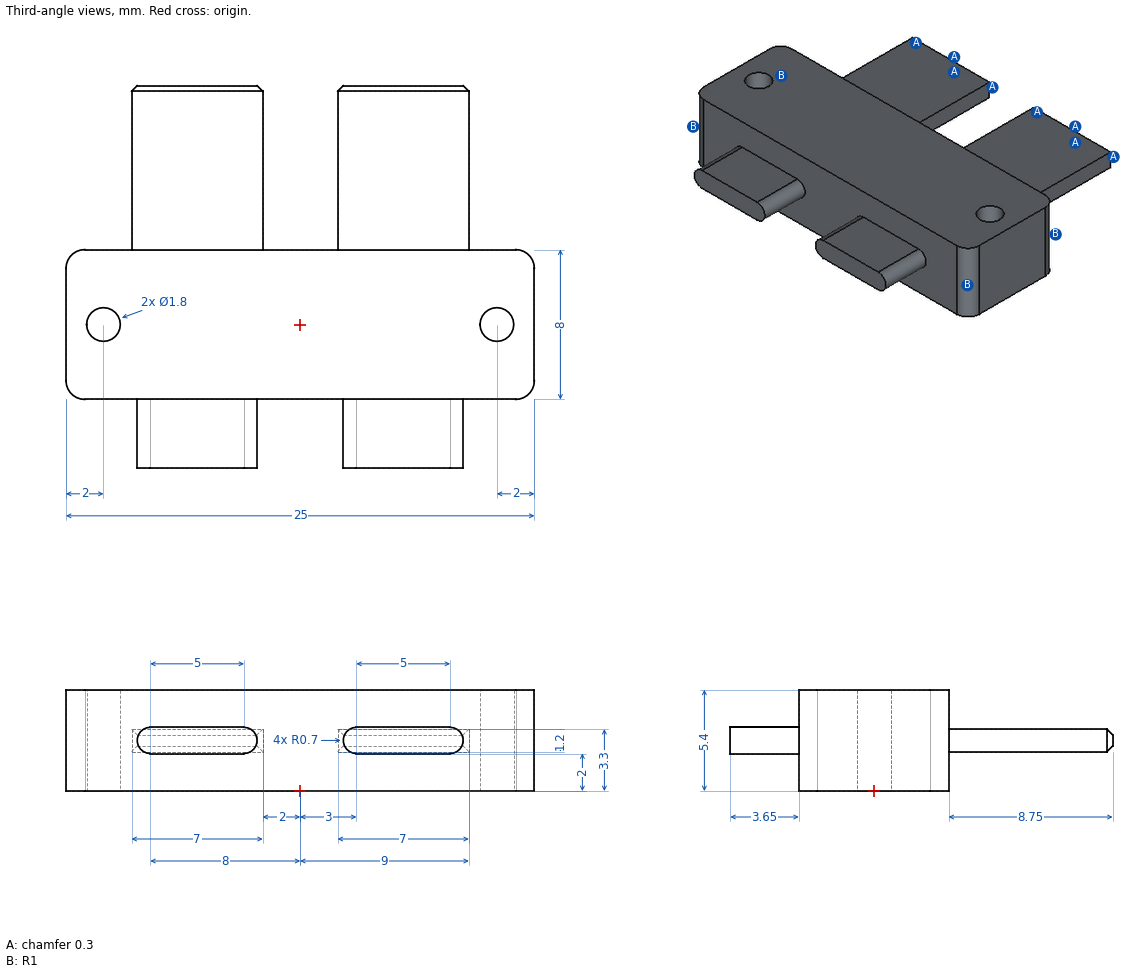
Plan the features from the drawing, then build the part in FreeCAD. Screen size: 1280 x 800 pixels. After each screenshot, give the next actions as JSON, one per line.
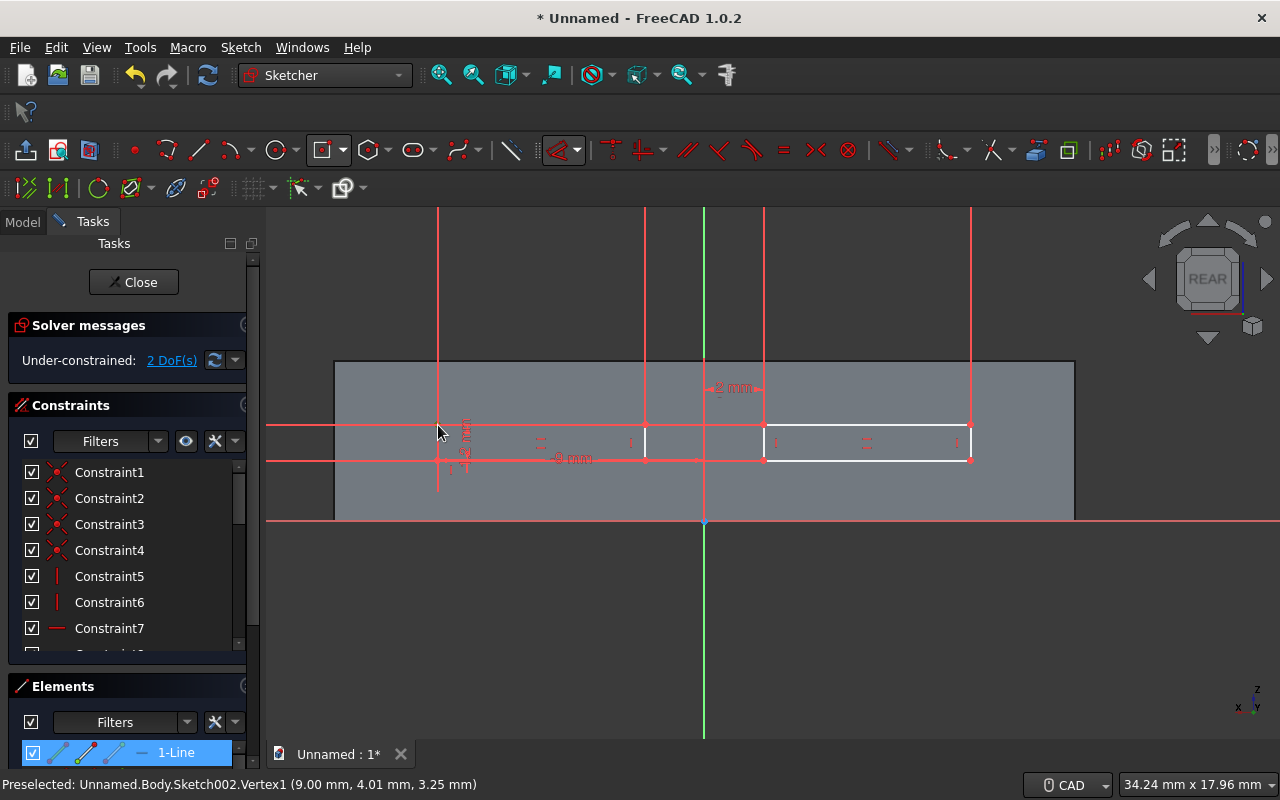
{"action": "key", "text": "i"}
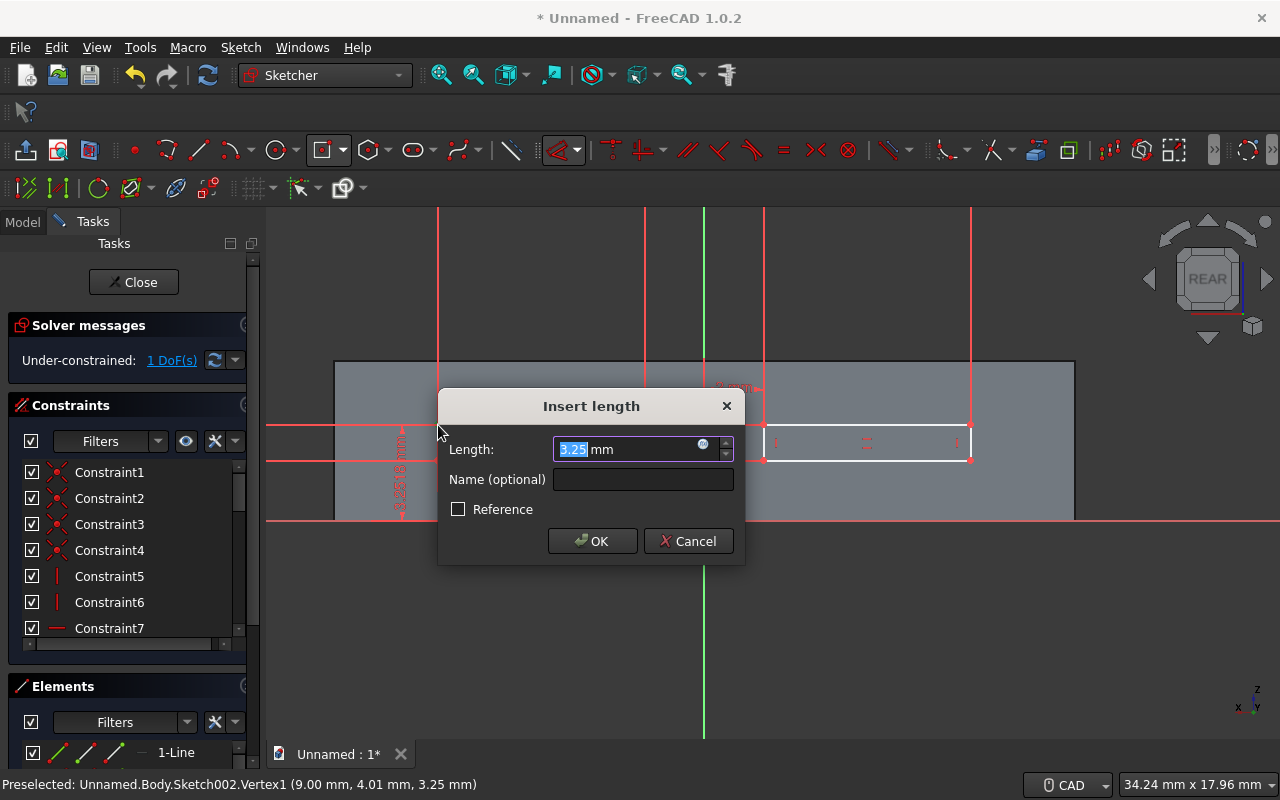
{"action": "type", "text": "3.3"}
{"action": "key", "text": "Return"}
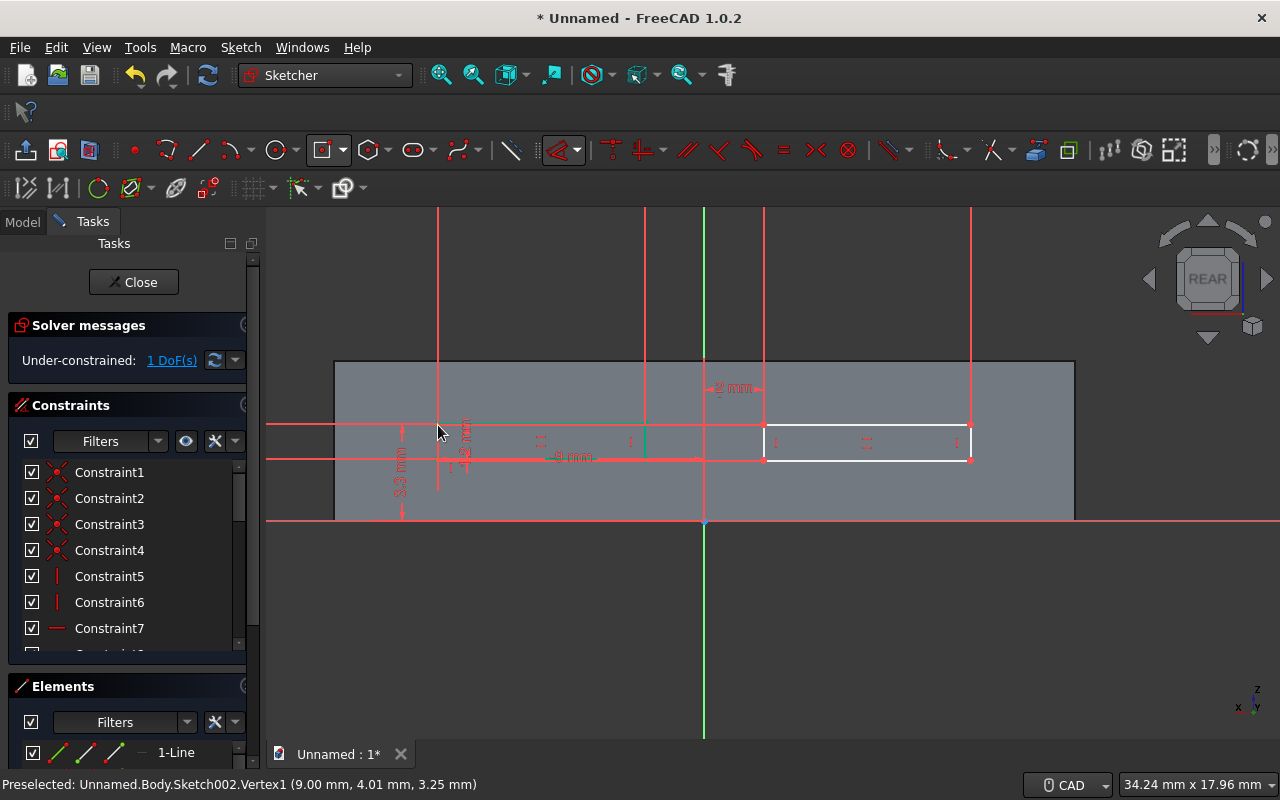
{"action": "left_click", "coordinate": [764, 425]}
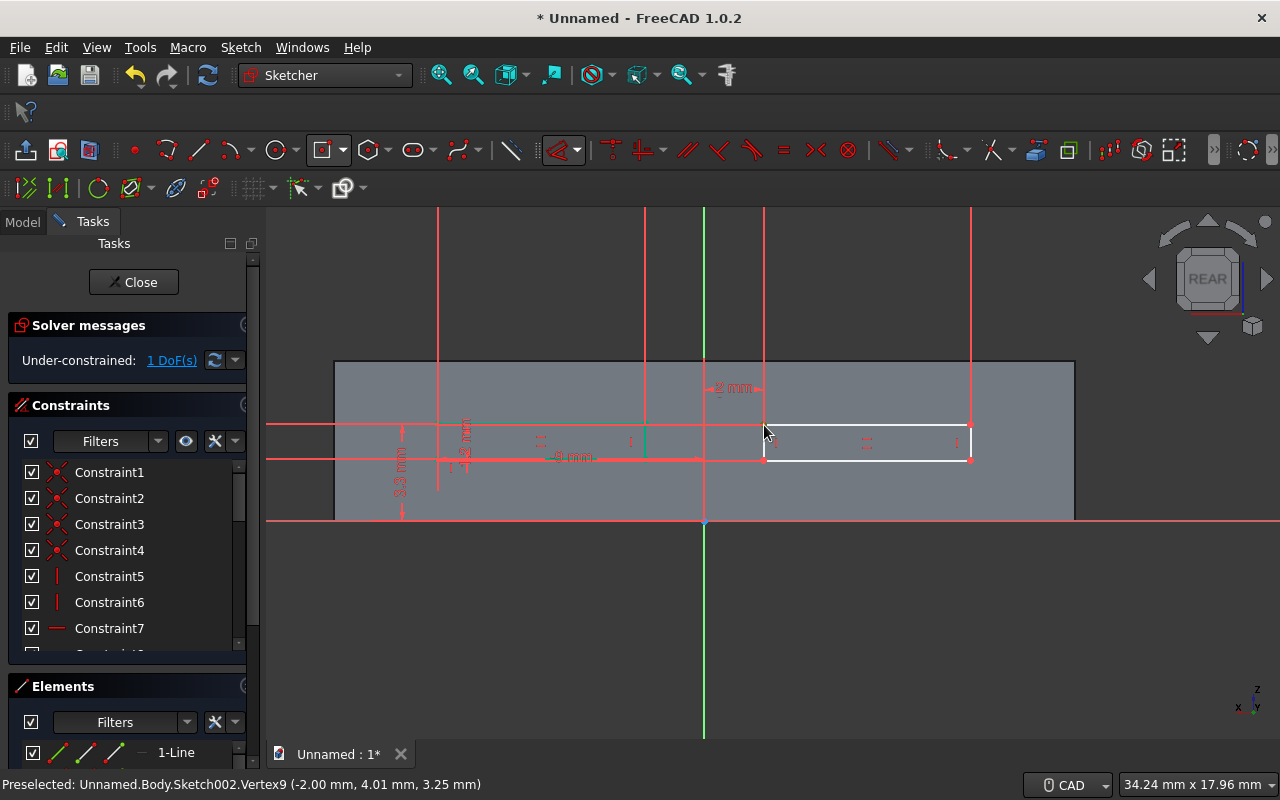
{"action": "left_click", "coordinate": [580, 150]}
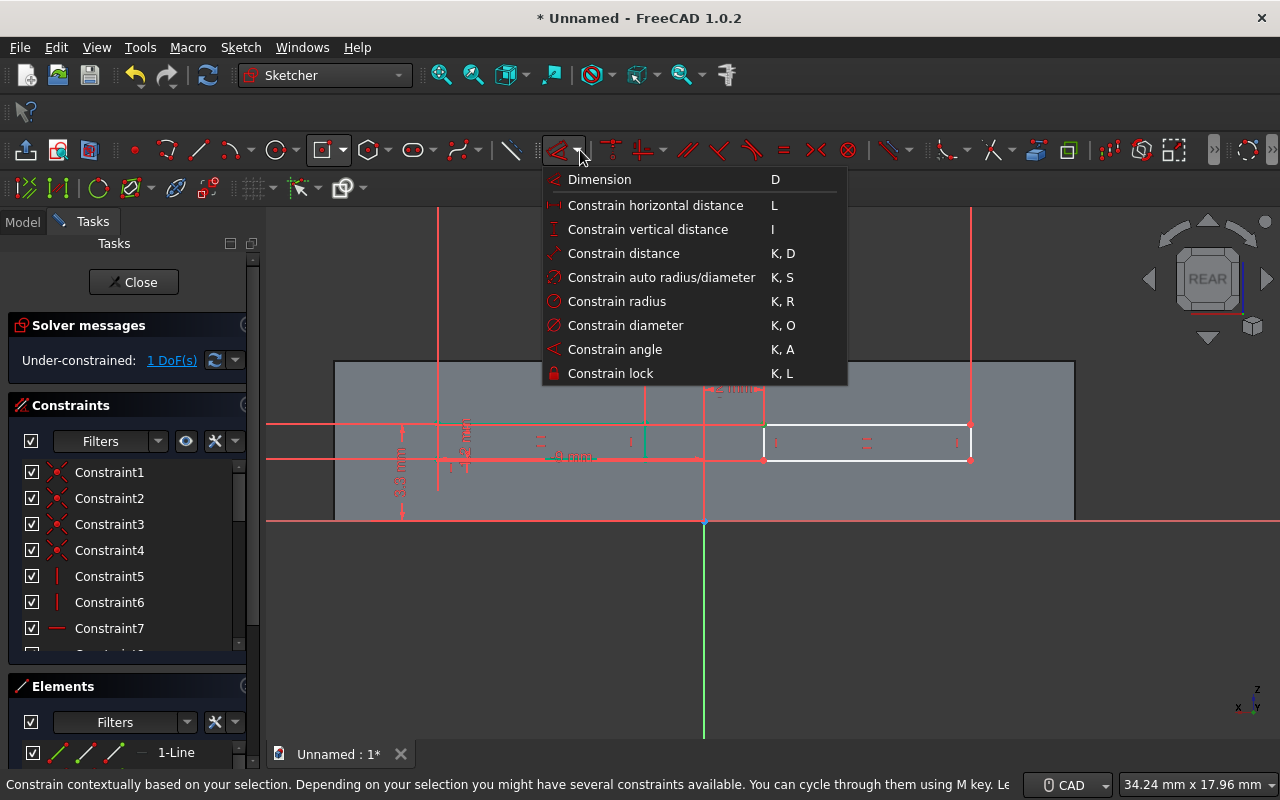
{"action": "left_click", "coordinate": [695, 229]}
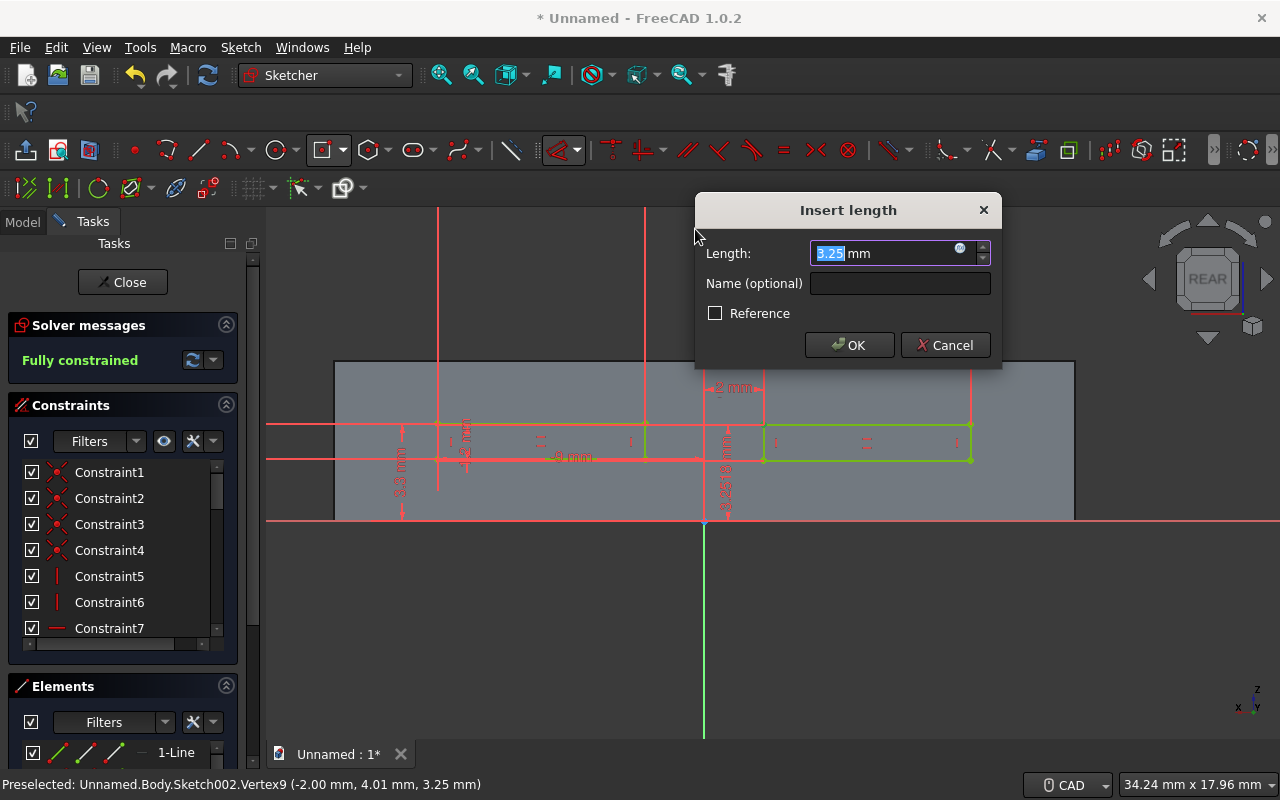
{"action": "type", "text": "3.3"}
{"action": "key", "text": "Return"}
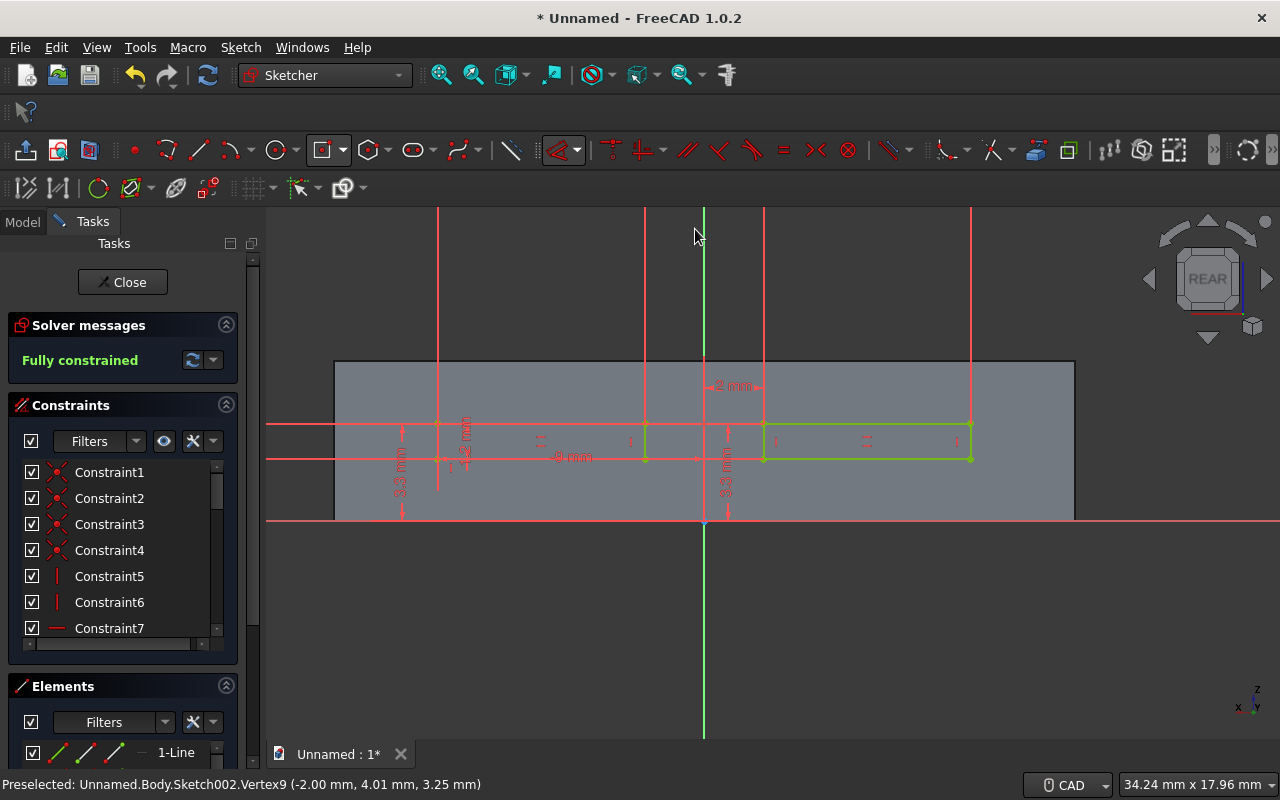
{"action": "left_click", "coordinate": [123, 282]}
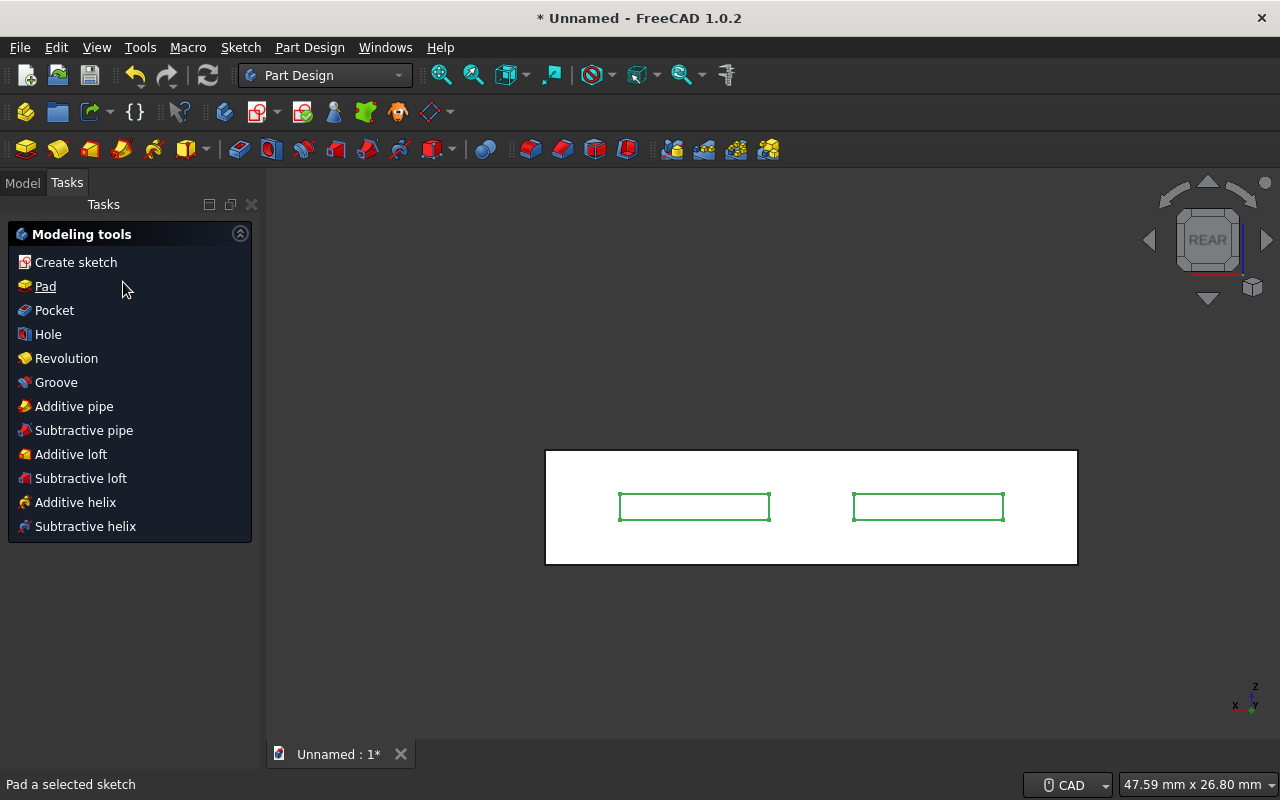
{"action": "left_click", "coordinate": [26, 150]}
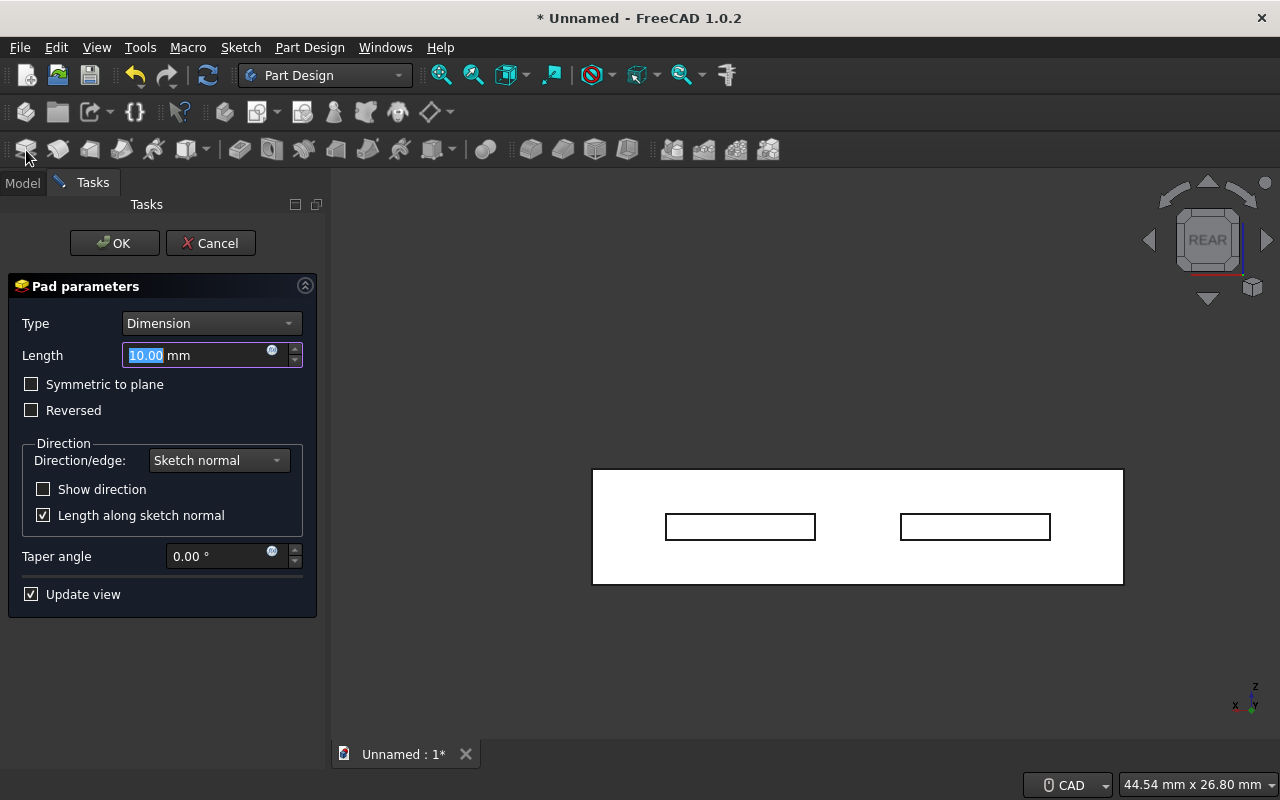
{"action": "type", "text": "8.75"}
{"action": "key", "text": "Tab"}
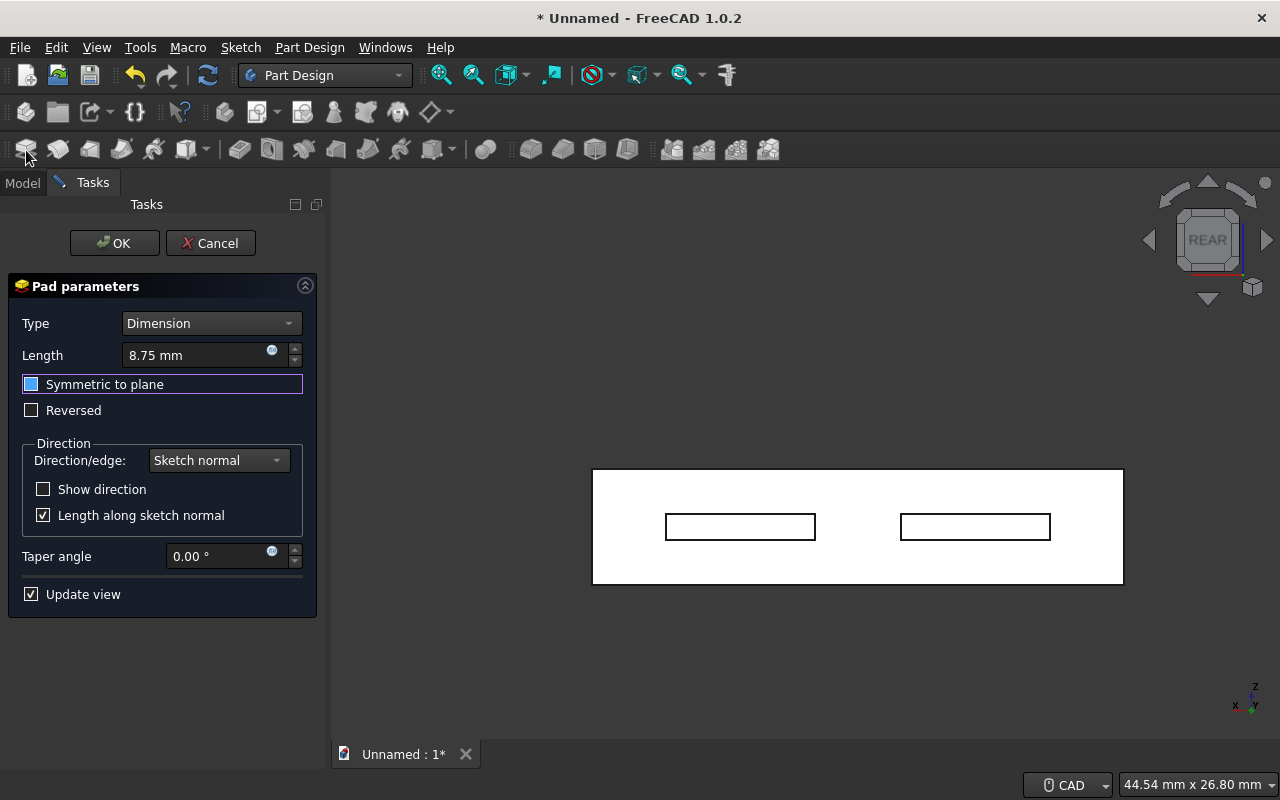
{"action": "left_click", "coordinate": [115, 243]}